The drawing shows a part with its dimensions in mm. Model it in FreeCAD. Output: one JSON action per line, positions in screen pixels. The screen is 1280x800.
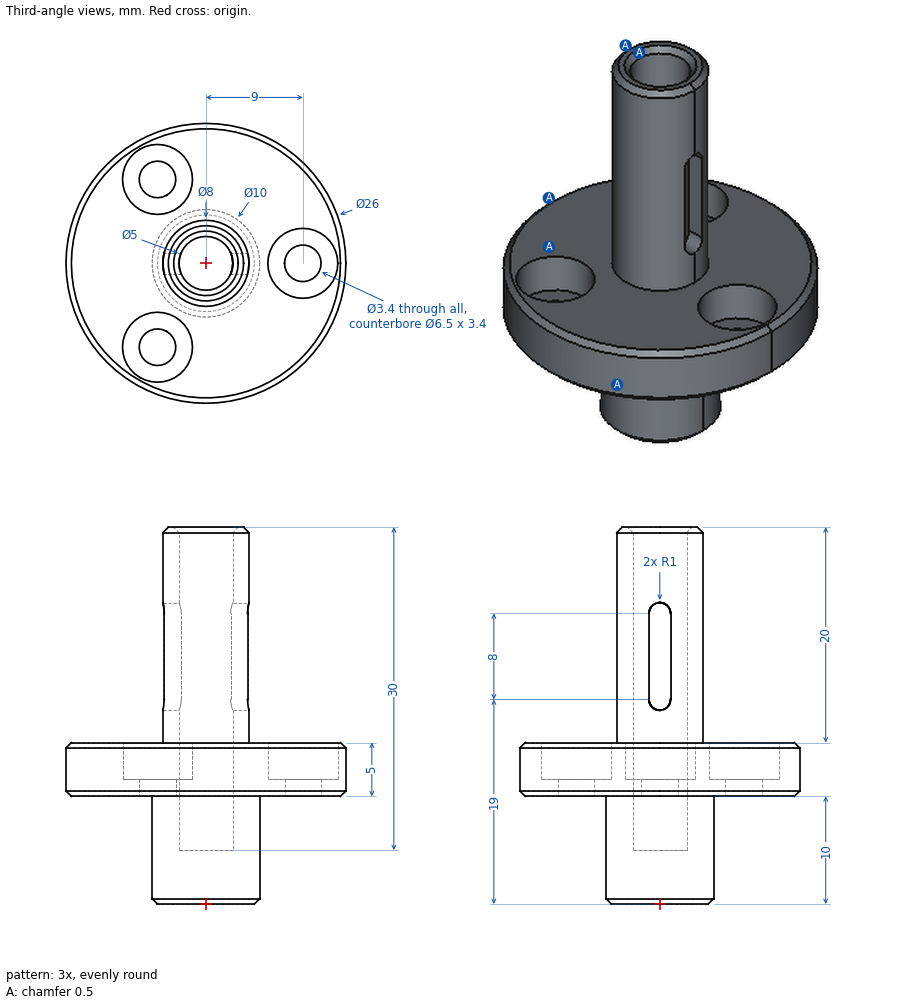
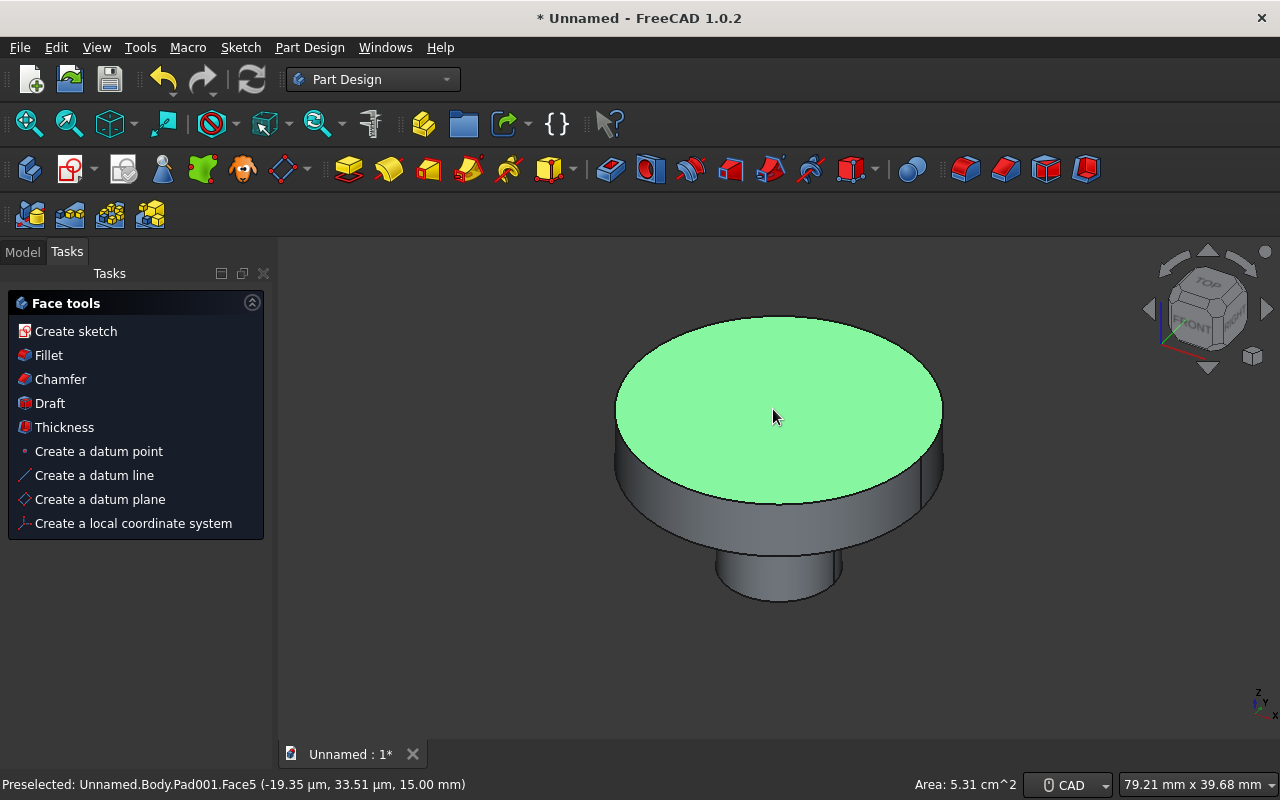
{"action": "left_click", "coordinate": [70, 170]}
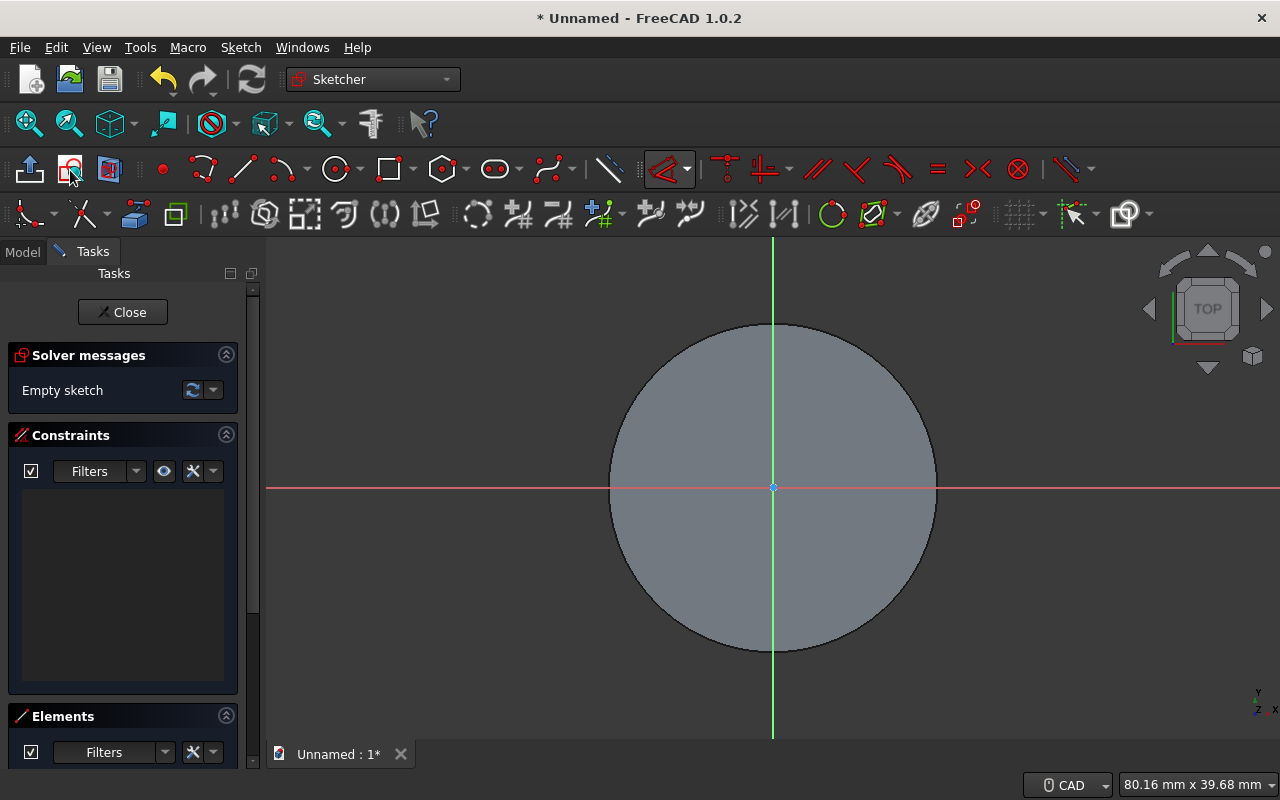
{"action": "scroll", "coordinate": [803, 488], "scroll_direction": "up", "scroll_amount": 6}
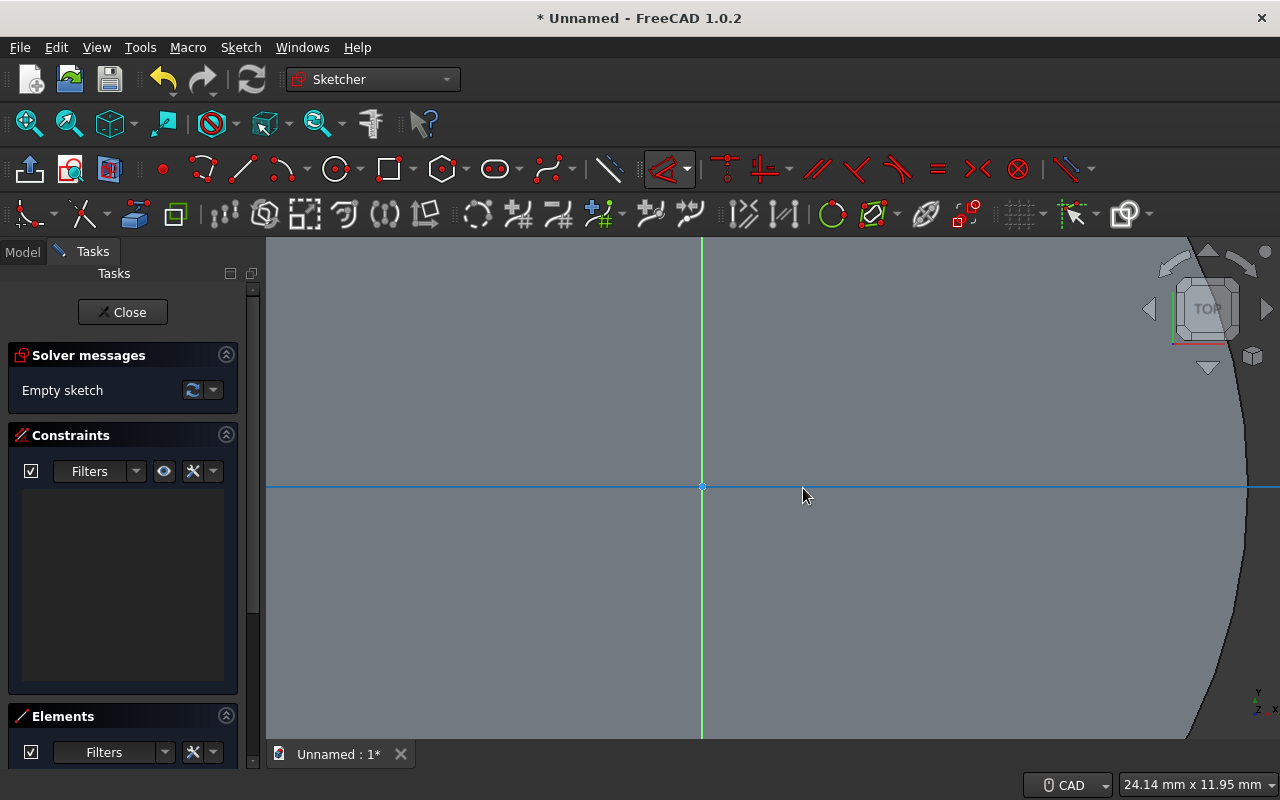
{"action": "left_click", "coordinate": [336, 170]}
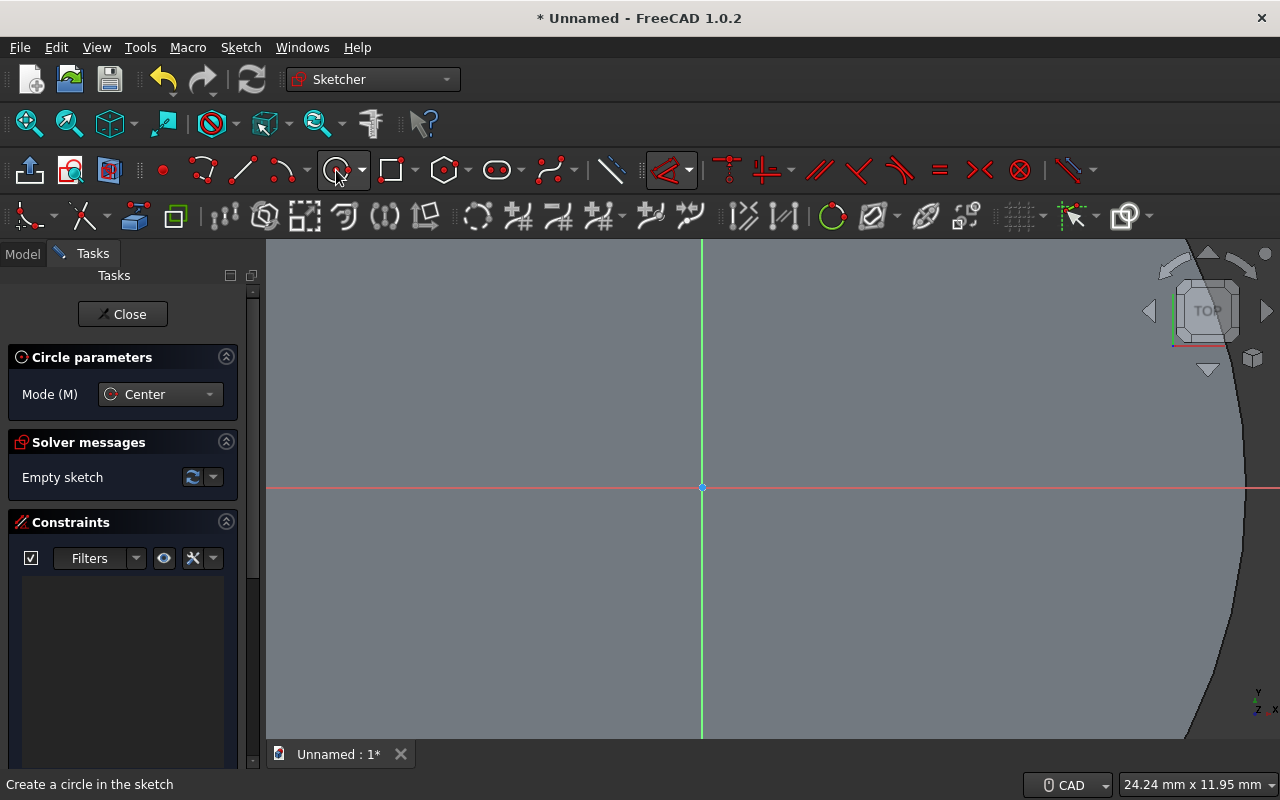
{"action": "left_click", "coordinate": [702, 488]}
{"action": "left_click", "coordinate": [821, 370]}
{"action": "key", "text": "Escape"}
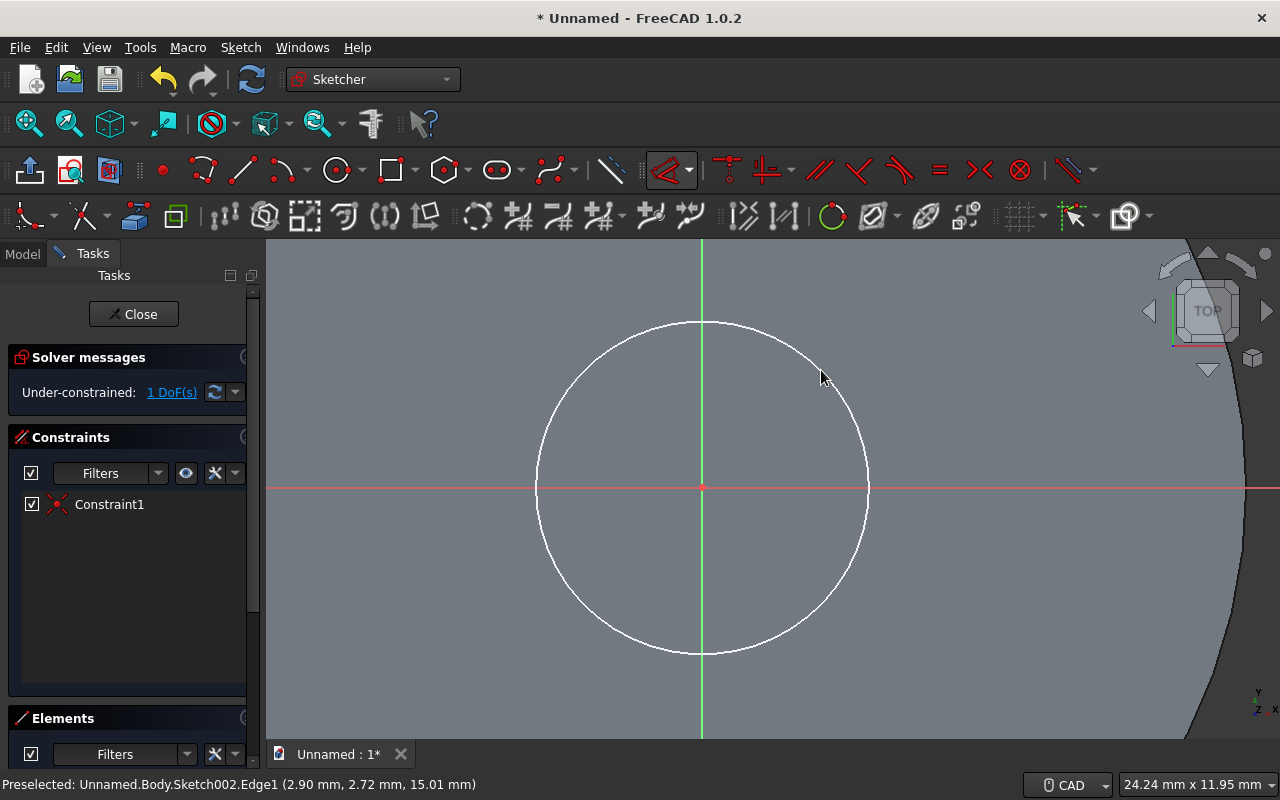
{"action": "left_click", "coordinate": [820, 370]}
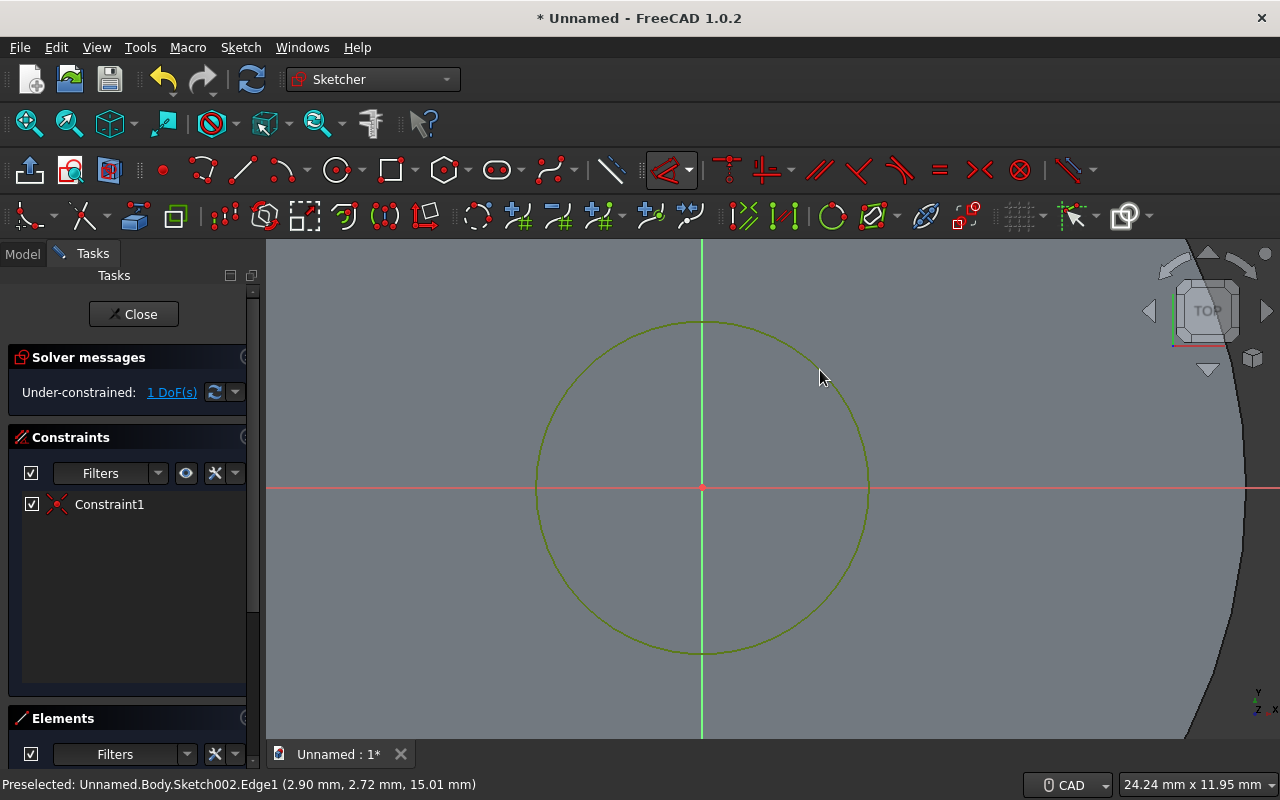
{"action": "key", "text": "k o"}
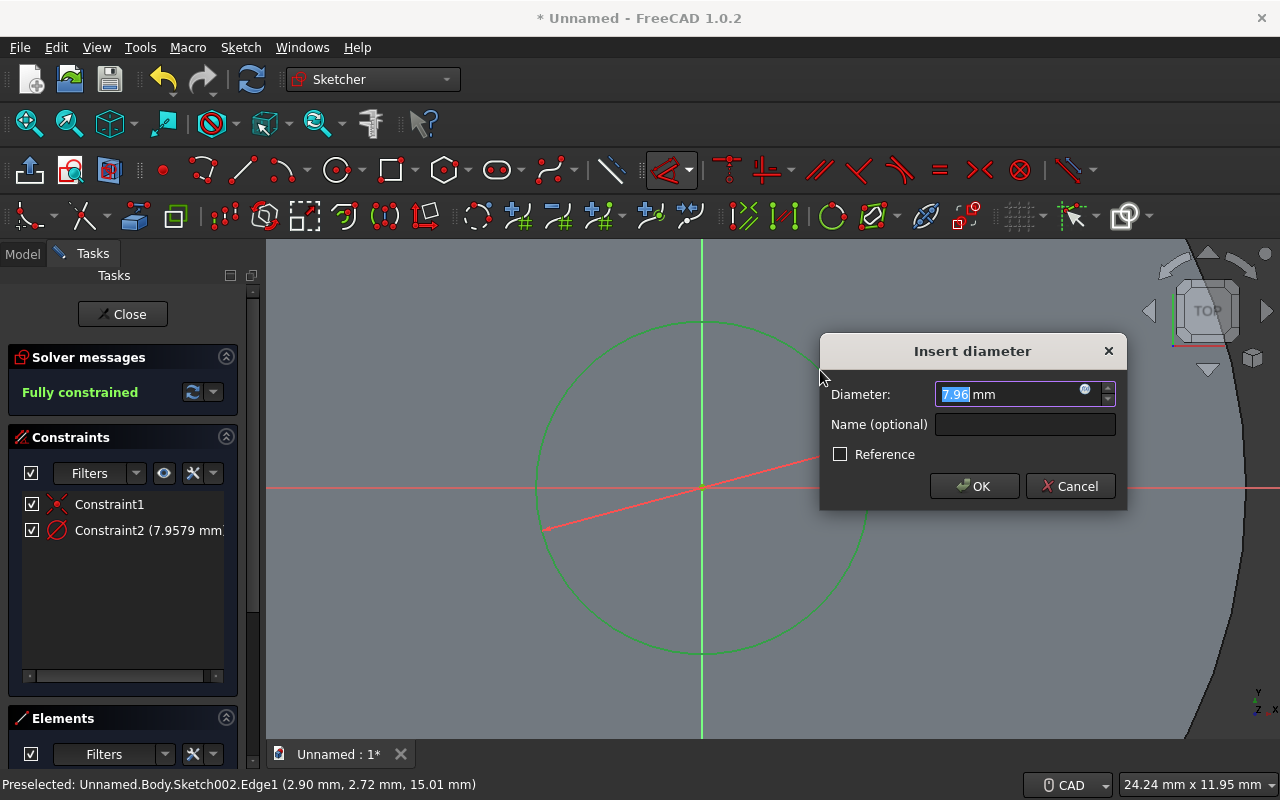
{"action": "type", "text": "8"}
{"action": "key", "text": "Return"}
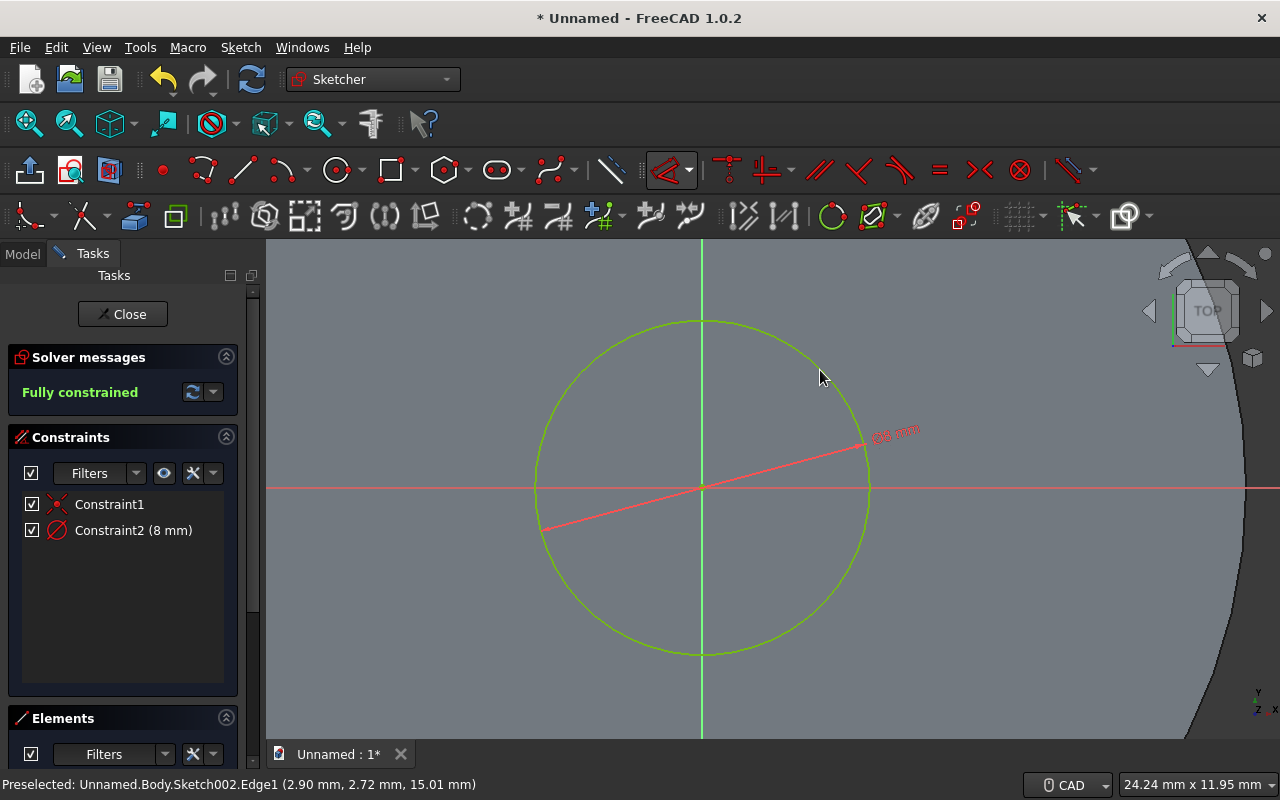
{"action": "left_click", "coordinate": [123, 314]}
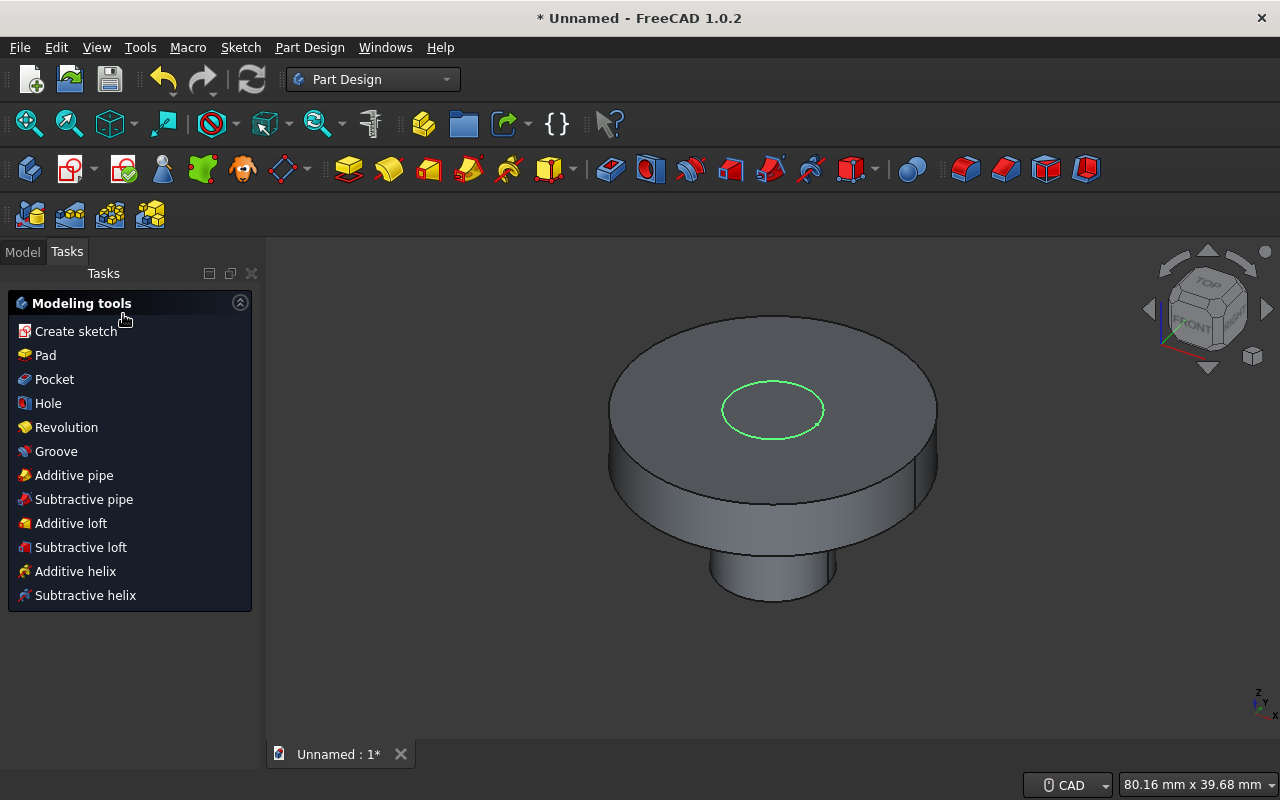
{"action": "left_click", "coordinate": [350, 170]}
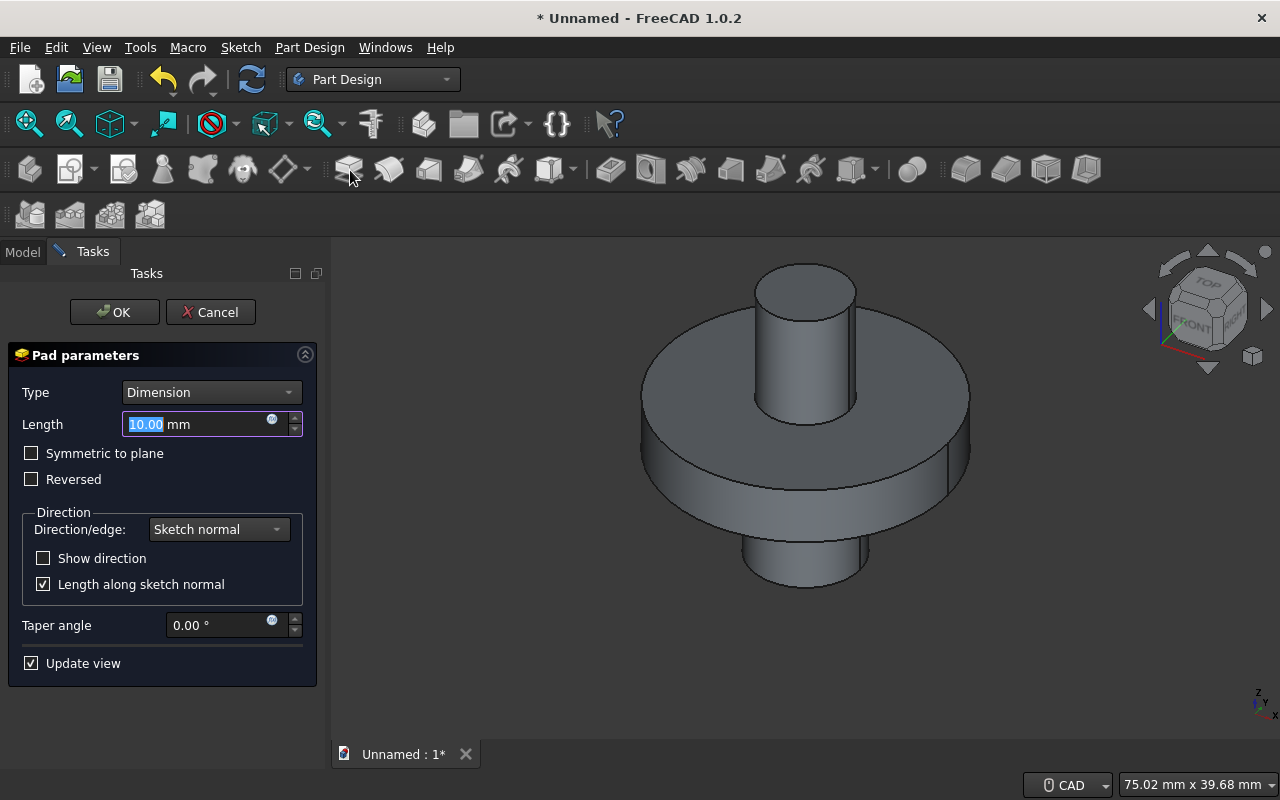
{"action": "type", "text": "20"}
{"action": "key", "text": "Tab"}